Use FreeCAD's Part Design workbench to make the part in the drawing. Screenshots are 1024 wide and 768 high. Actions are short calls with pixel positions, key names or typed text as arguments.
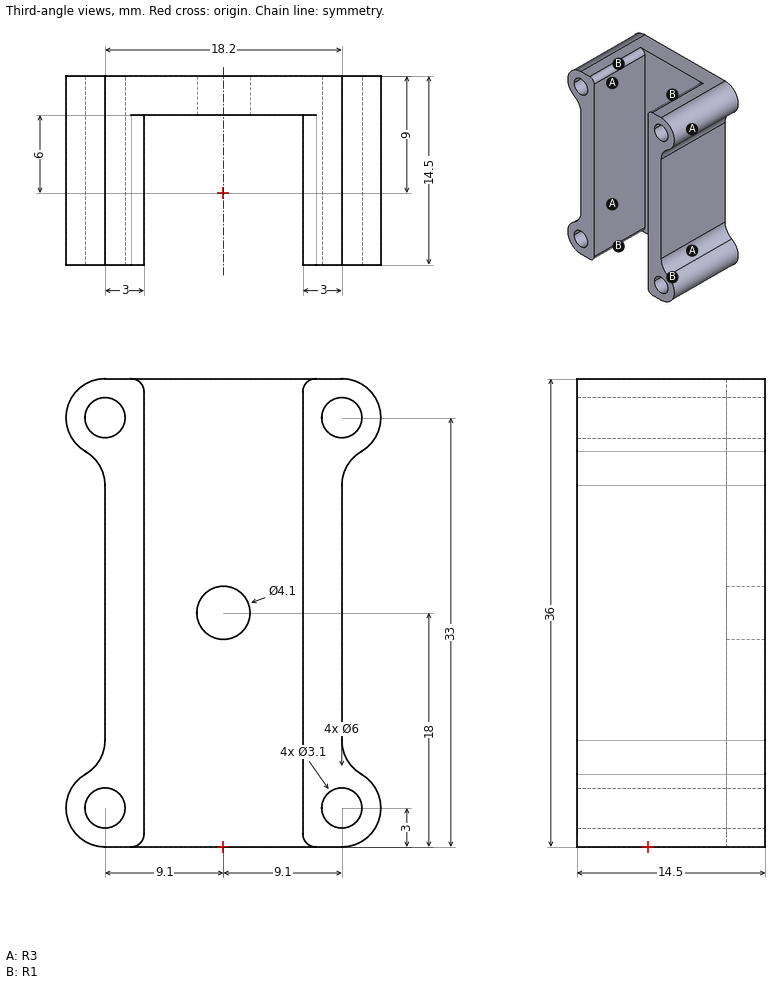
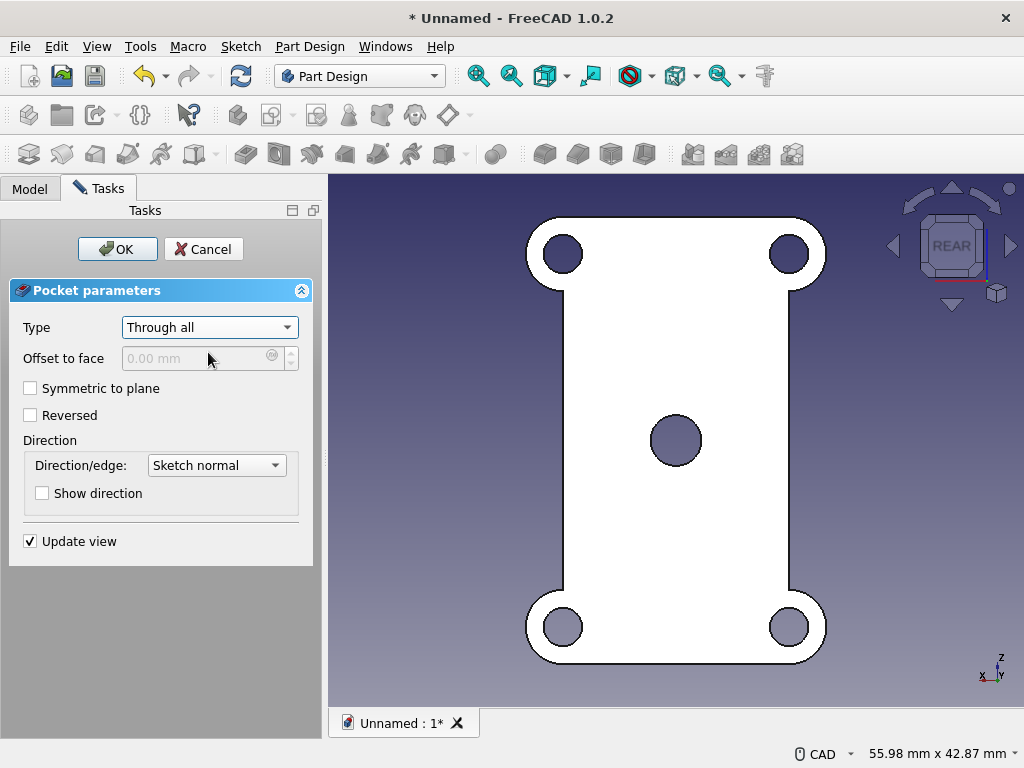
click(118, 249)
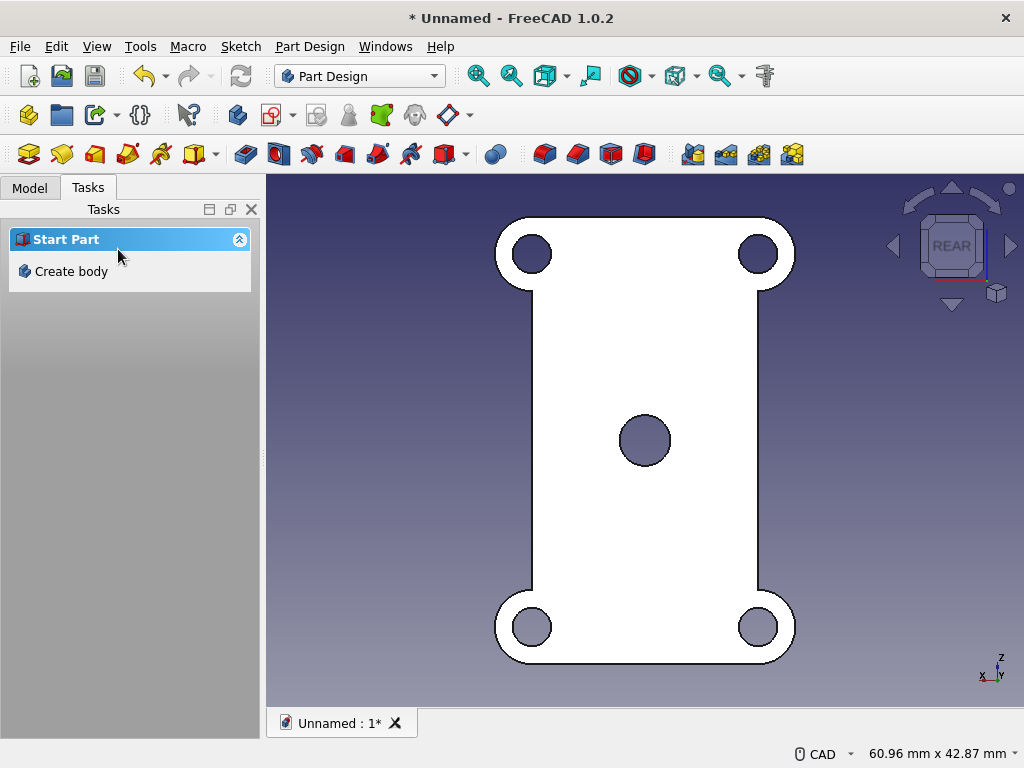
key(0)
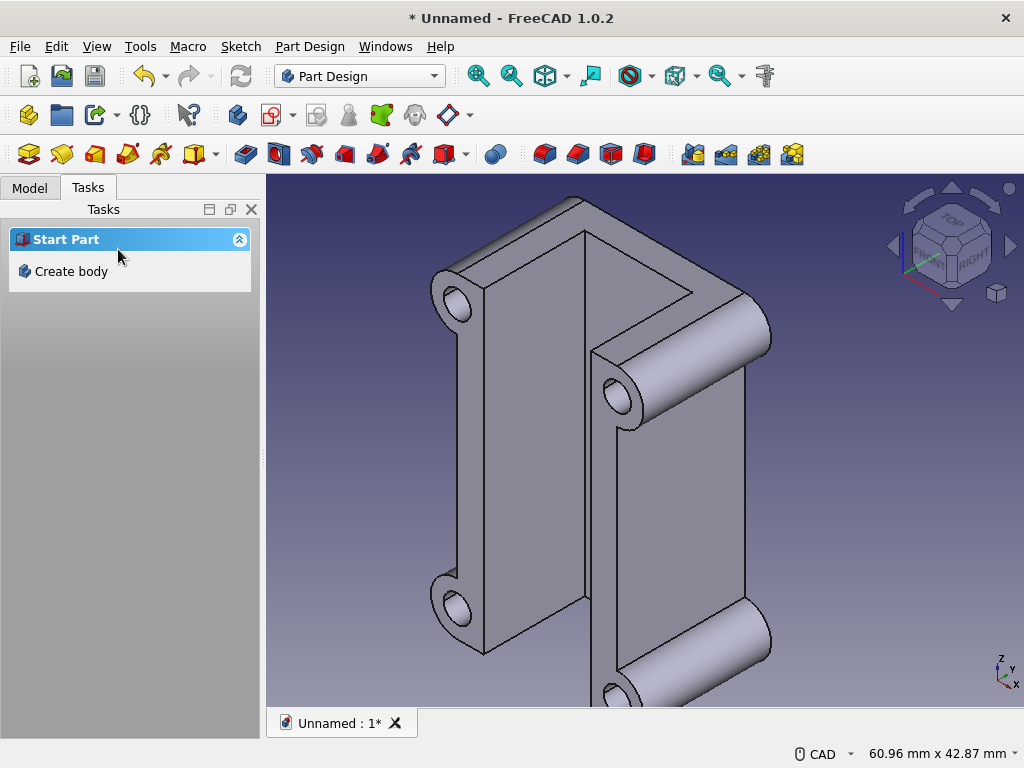
click(479, 76)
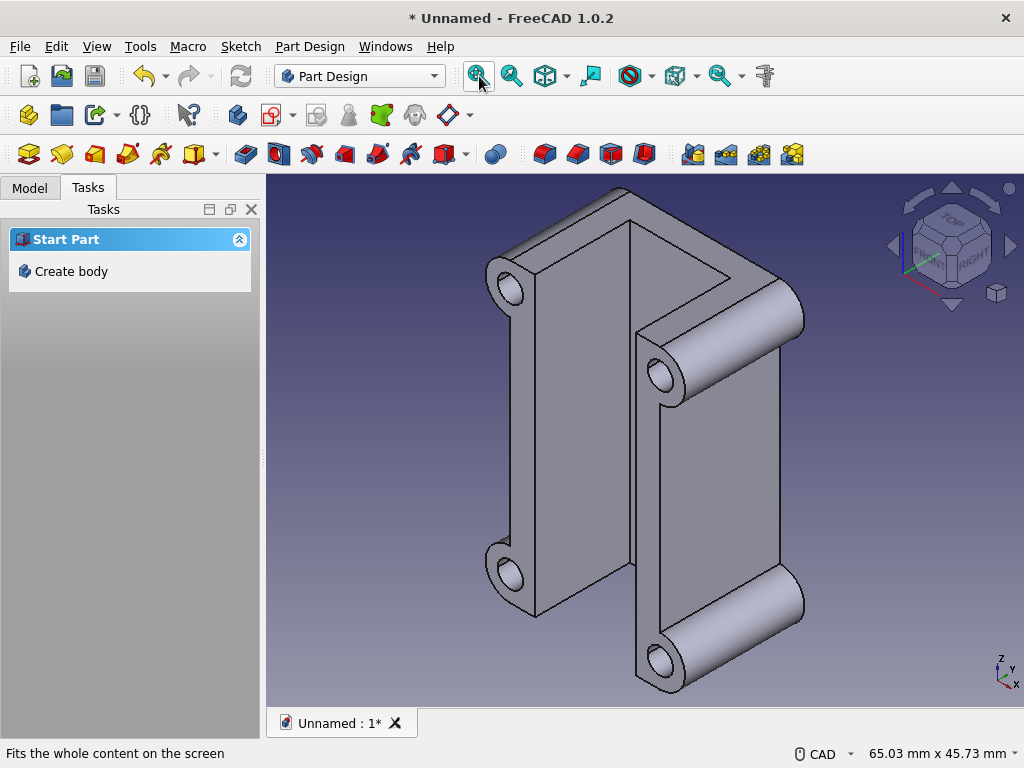
key(2)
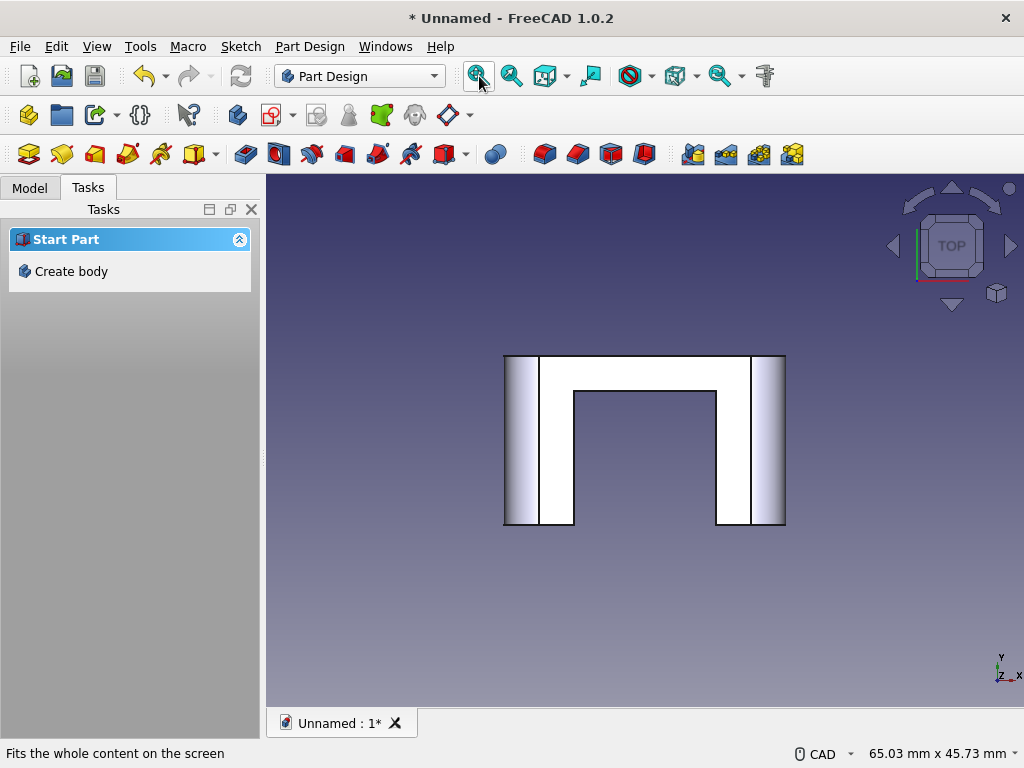
click(479, 76)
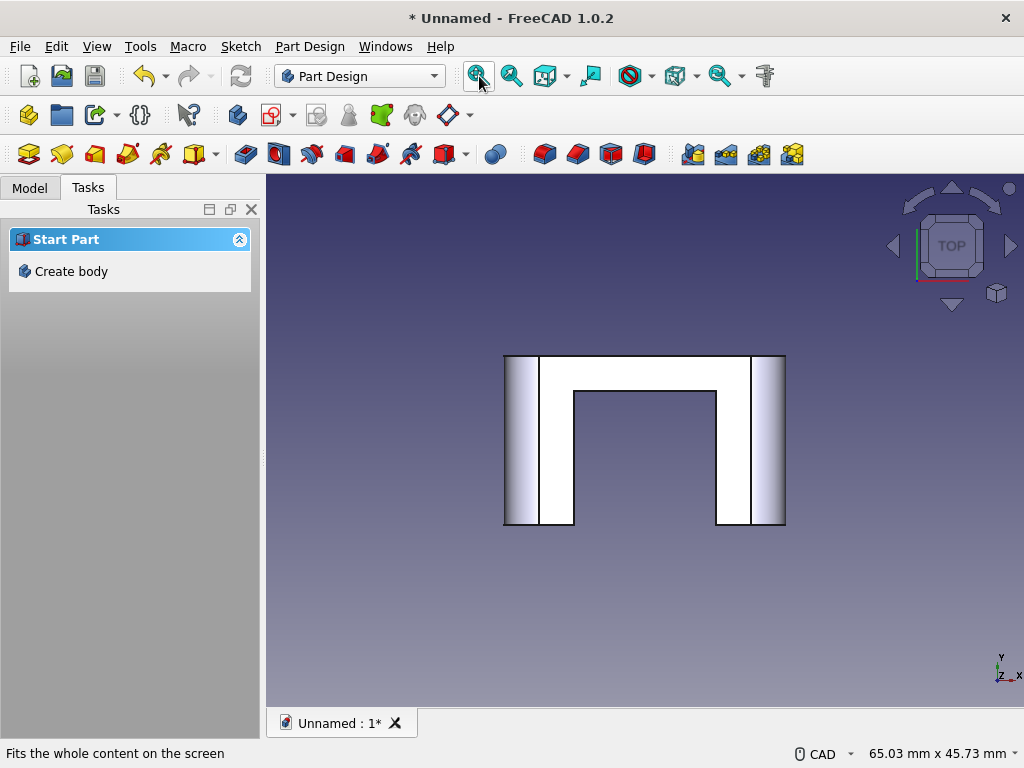
key(1)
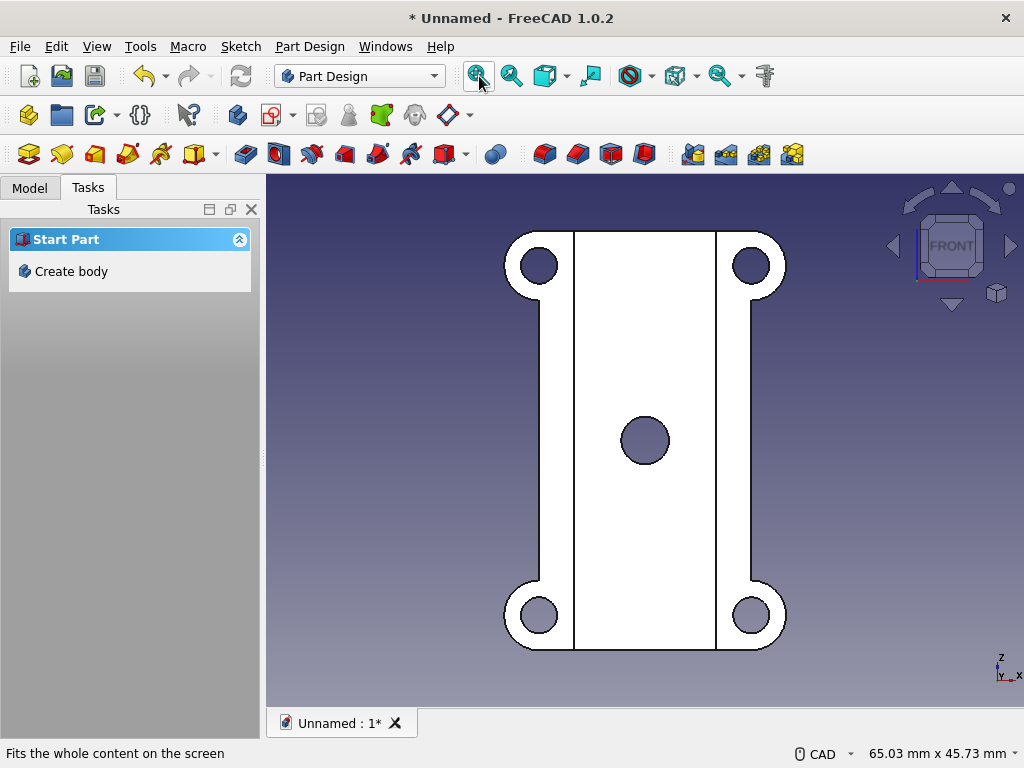
key(3)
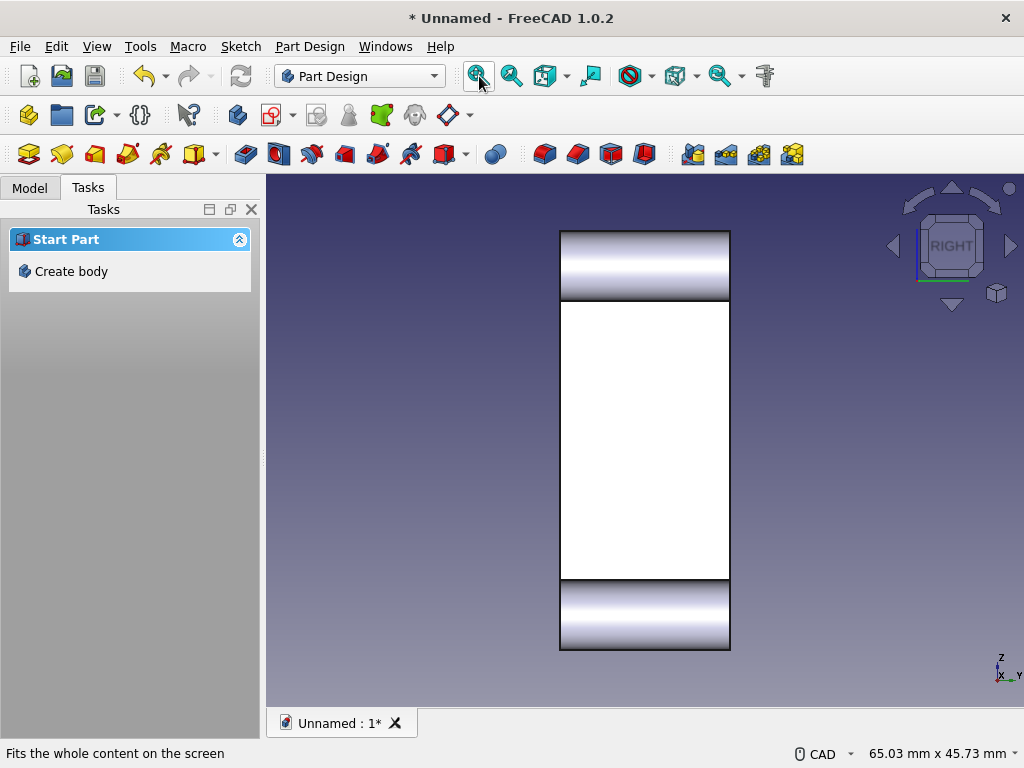
key(5)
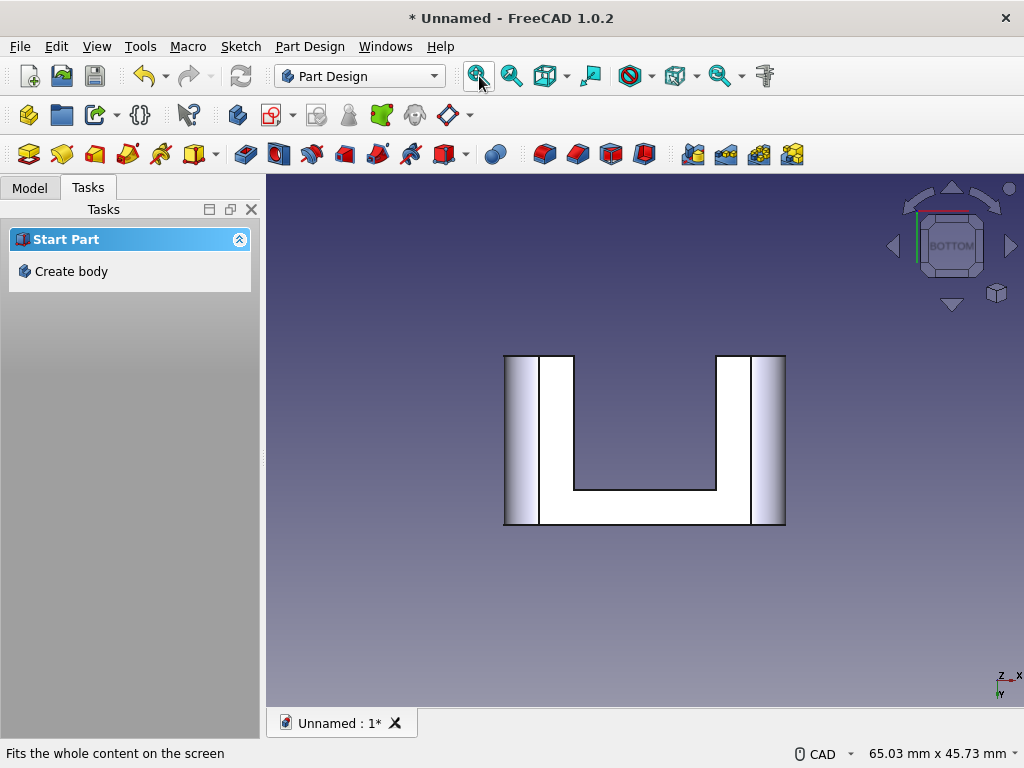
click(479, 76)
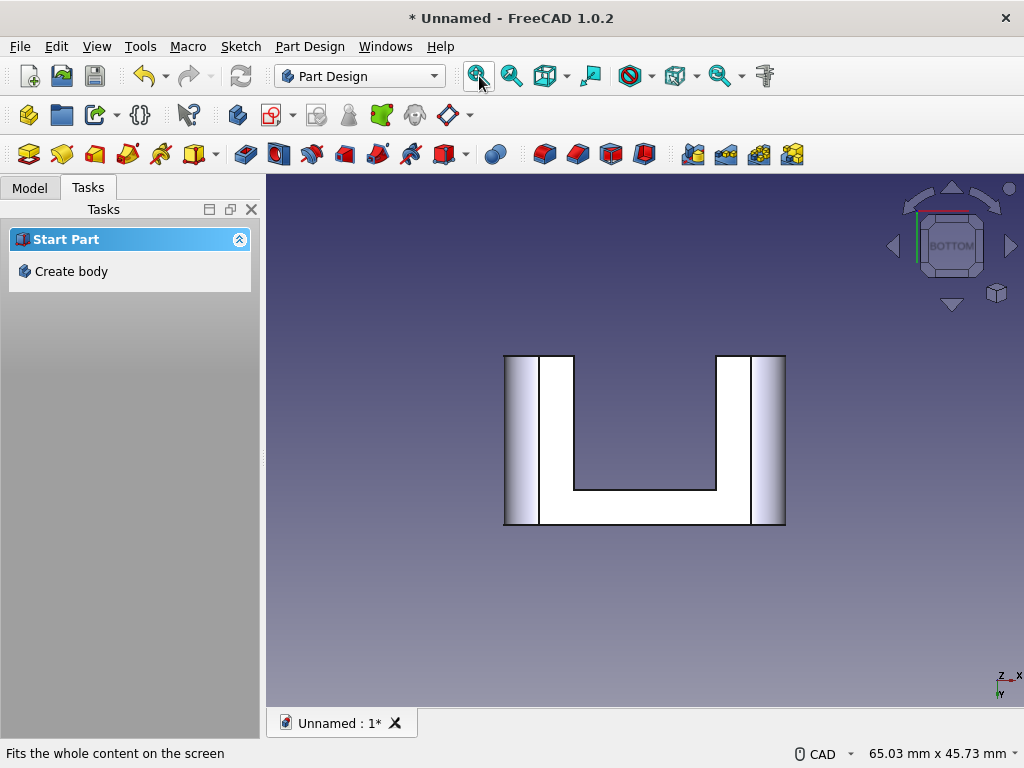
key(4)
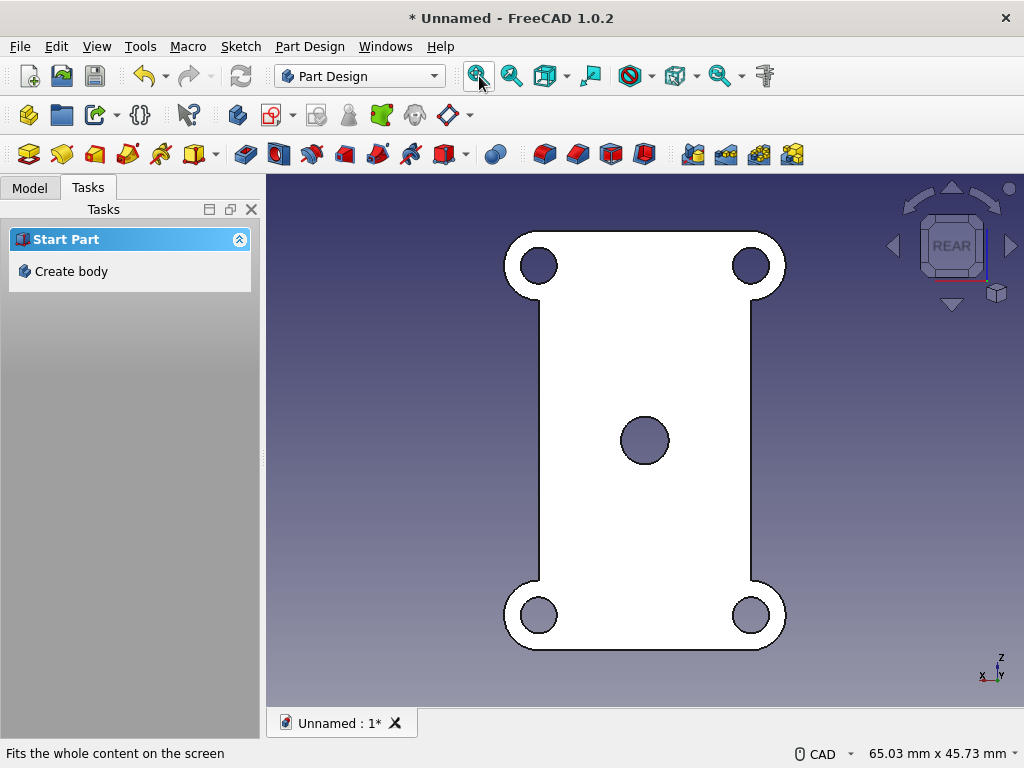
key(6)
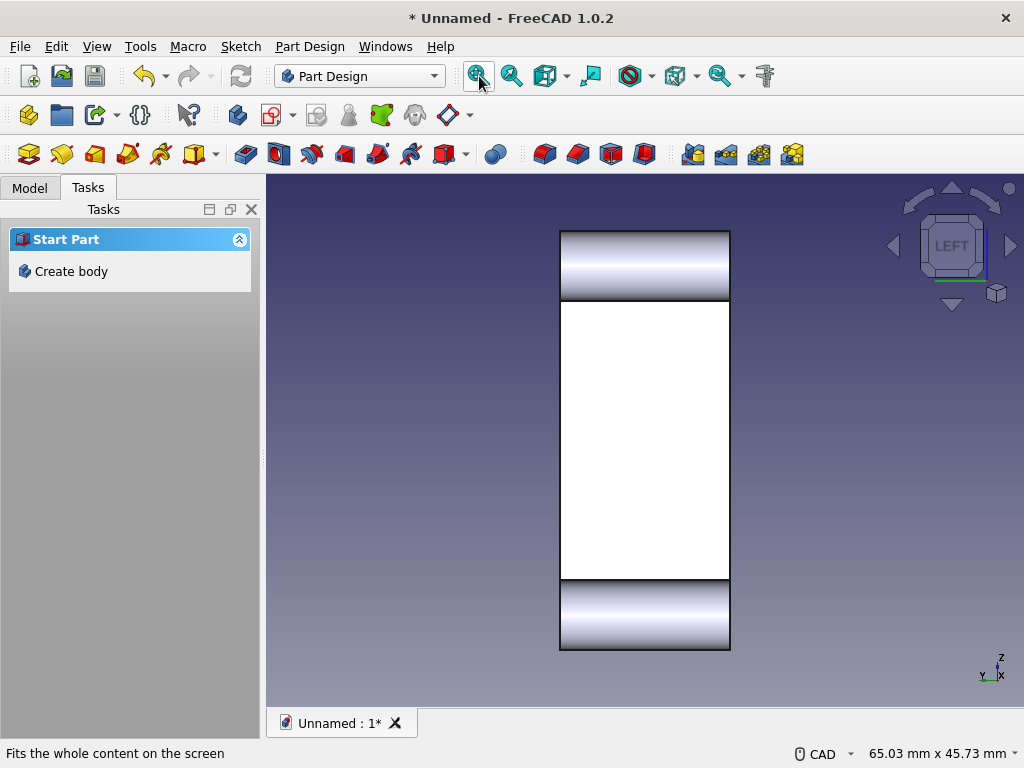
key(v)
key(3)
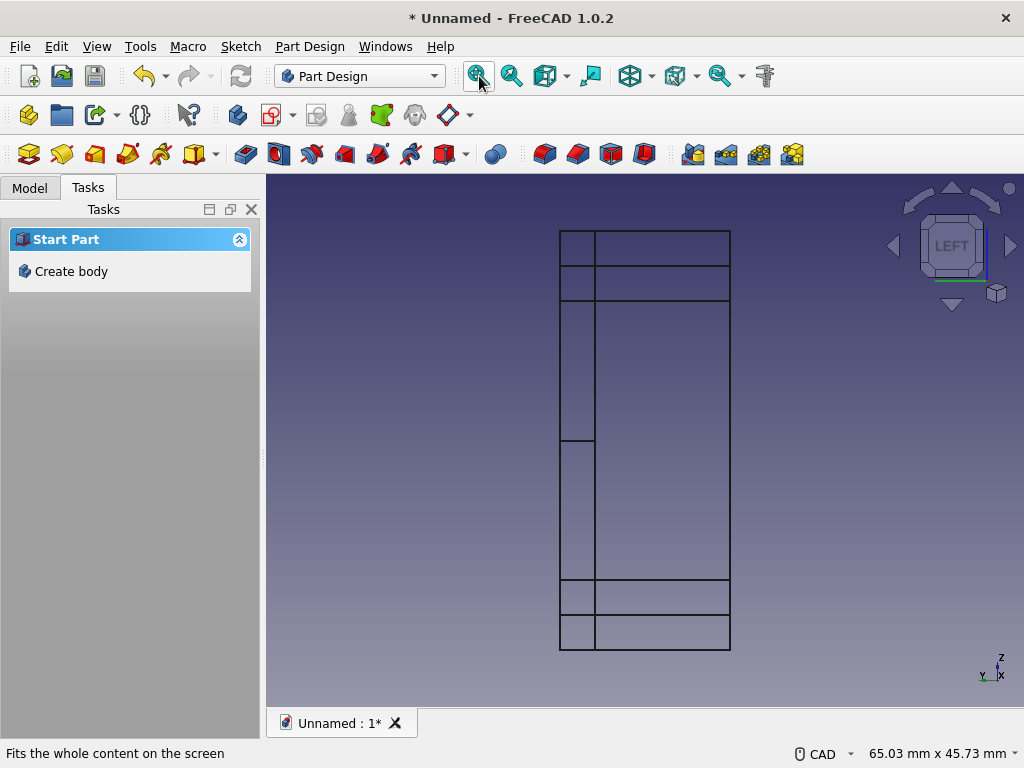
key(0)